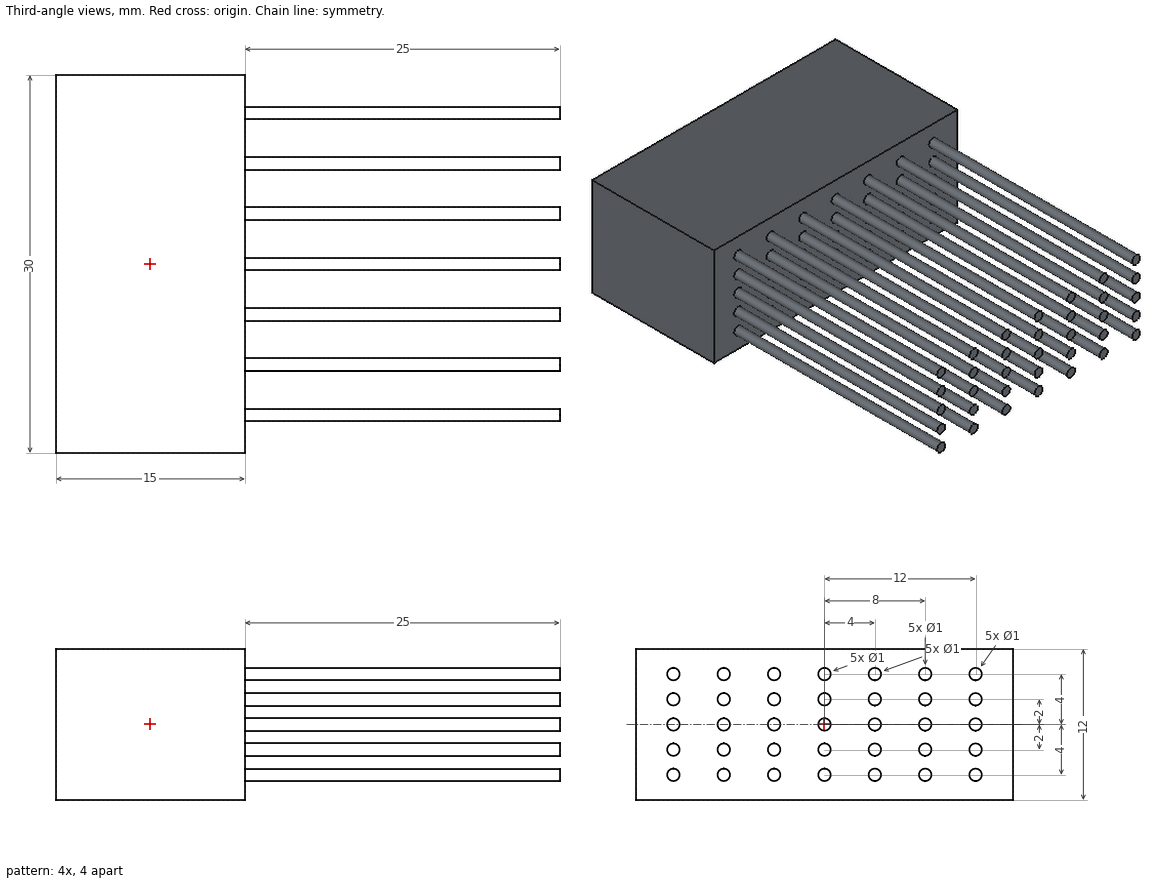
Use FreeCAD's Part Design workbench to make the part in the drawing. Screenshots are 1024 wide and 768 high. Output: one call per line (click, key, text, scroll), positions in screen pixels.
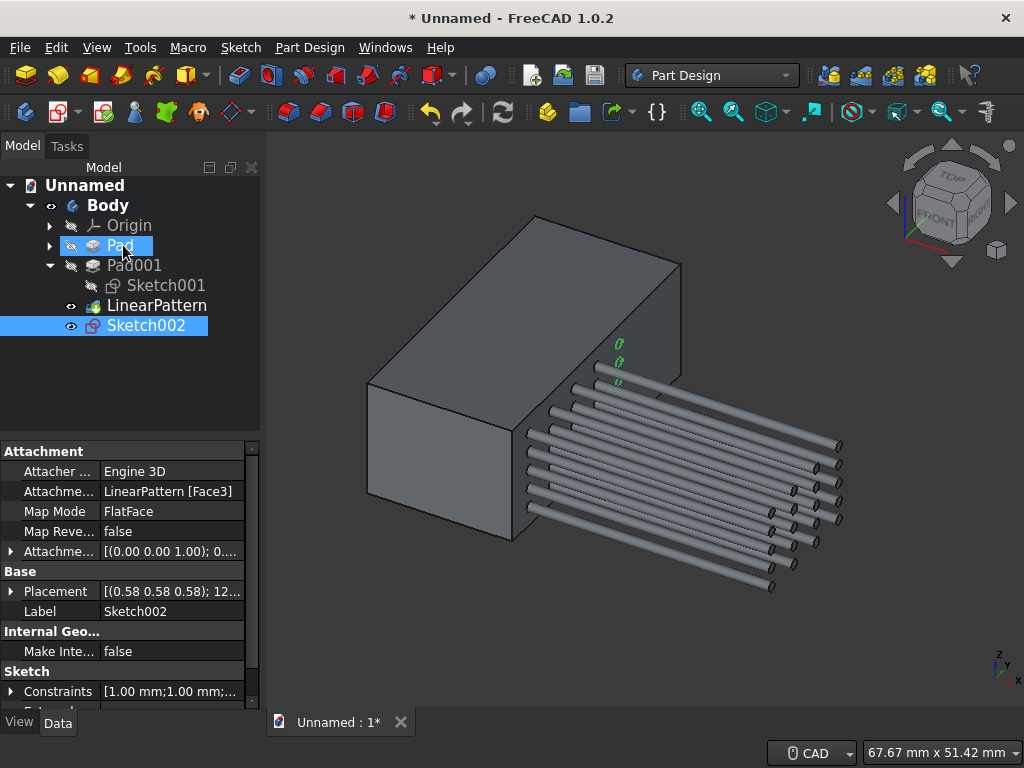
click(26, 76)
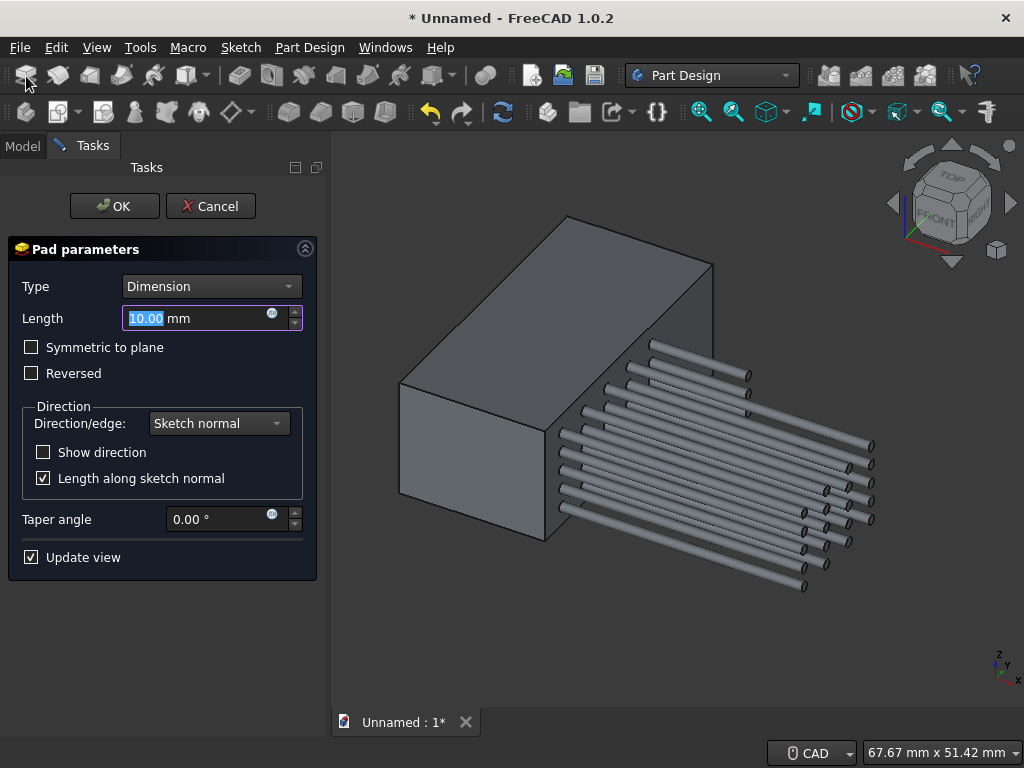
text(25)
key(Tab)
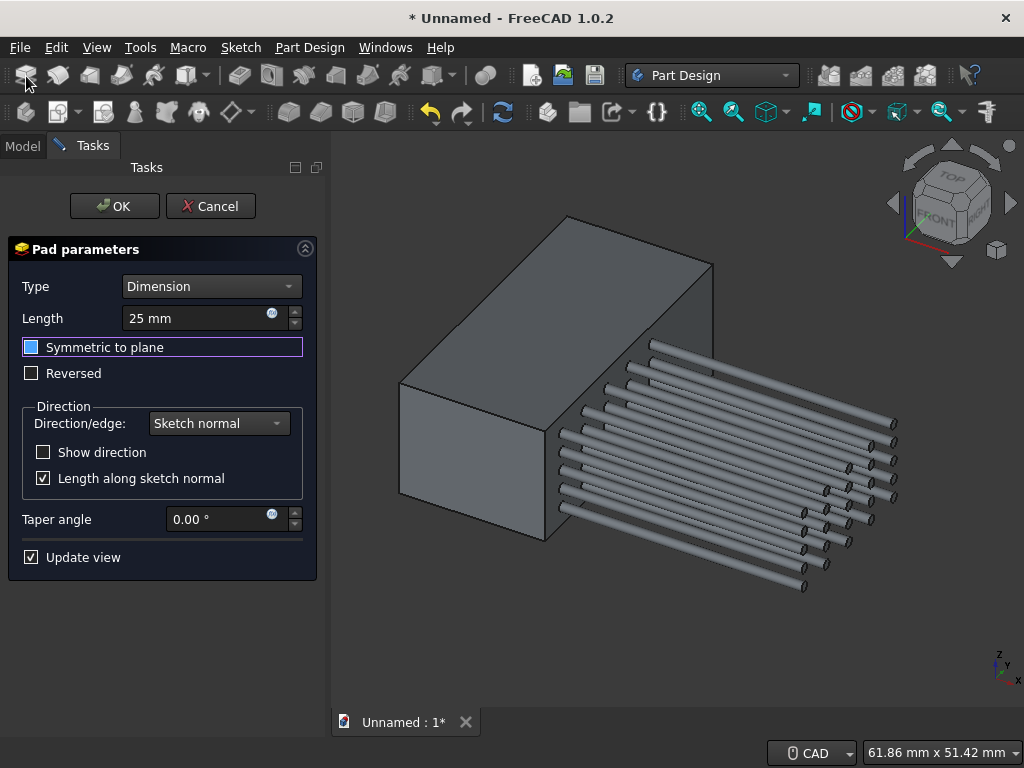
click(115, 206)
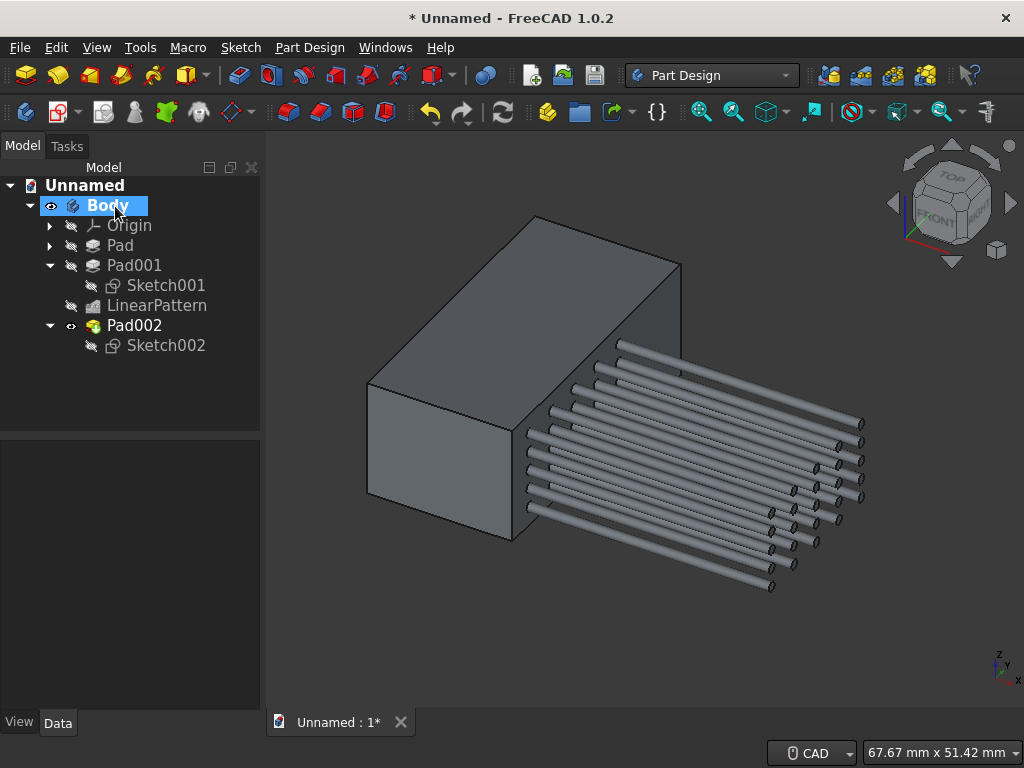
click(645, 323)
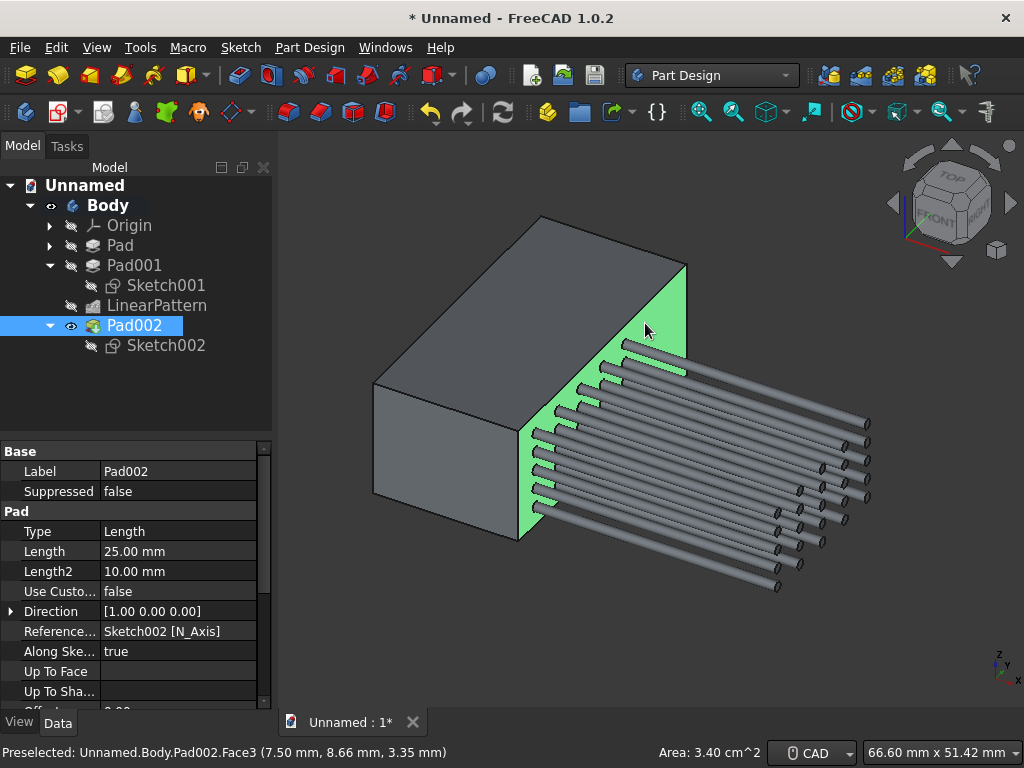
click(58, 112)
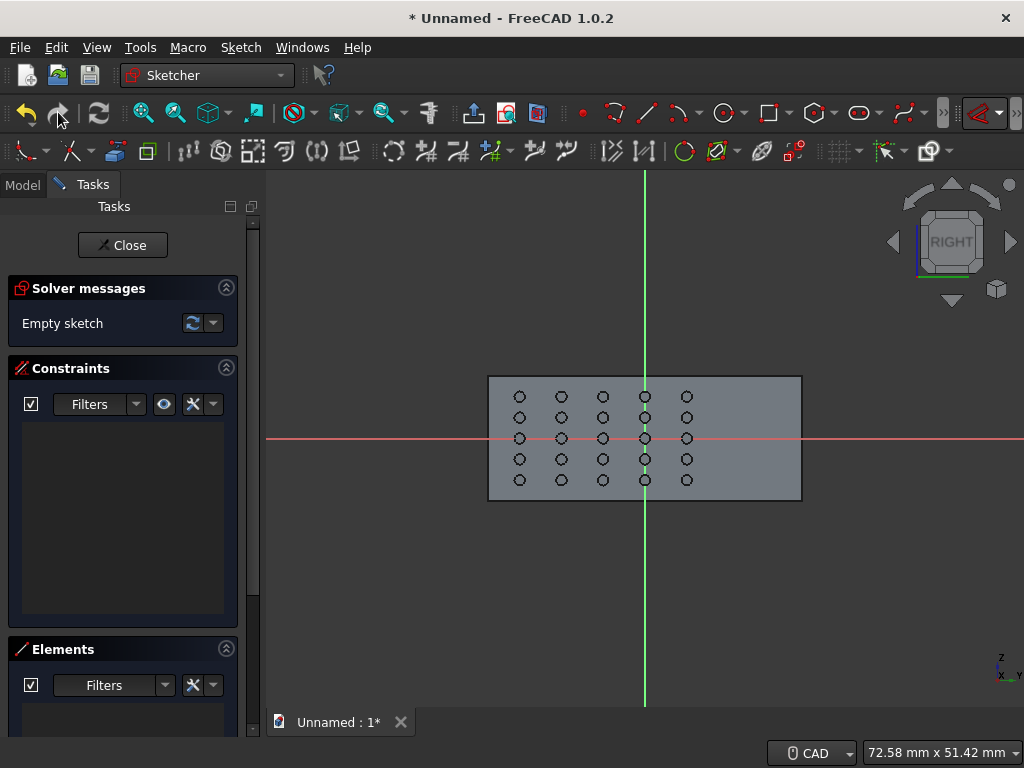
scroll(738, 438, up, 6)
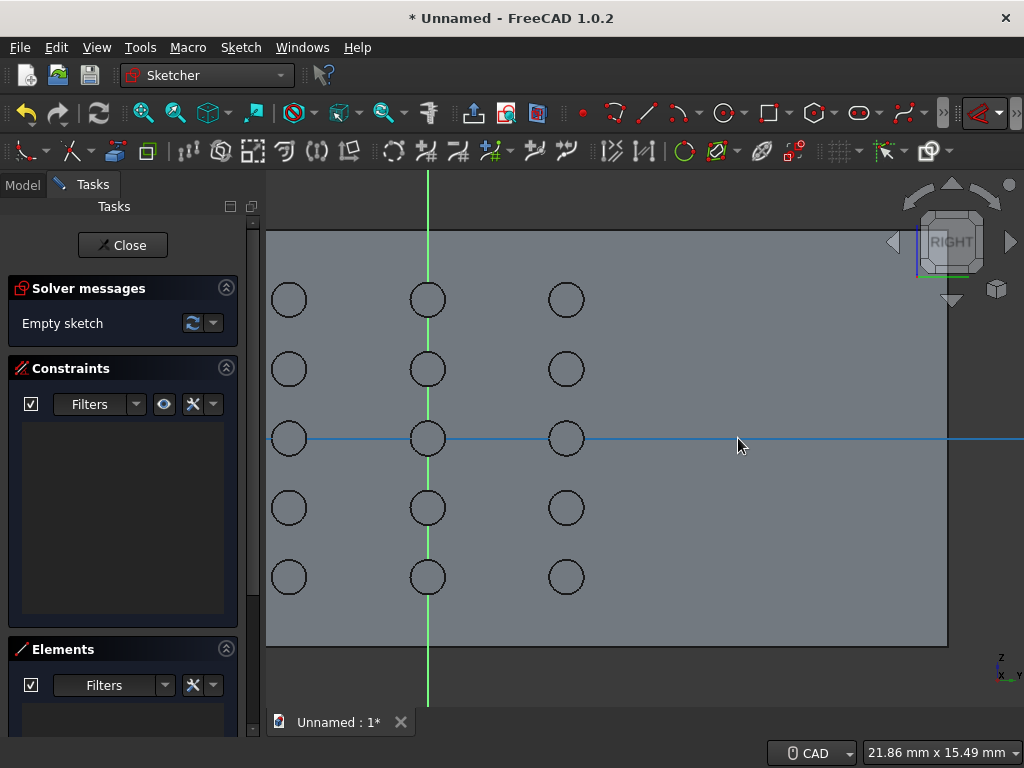
click(724, 114)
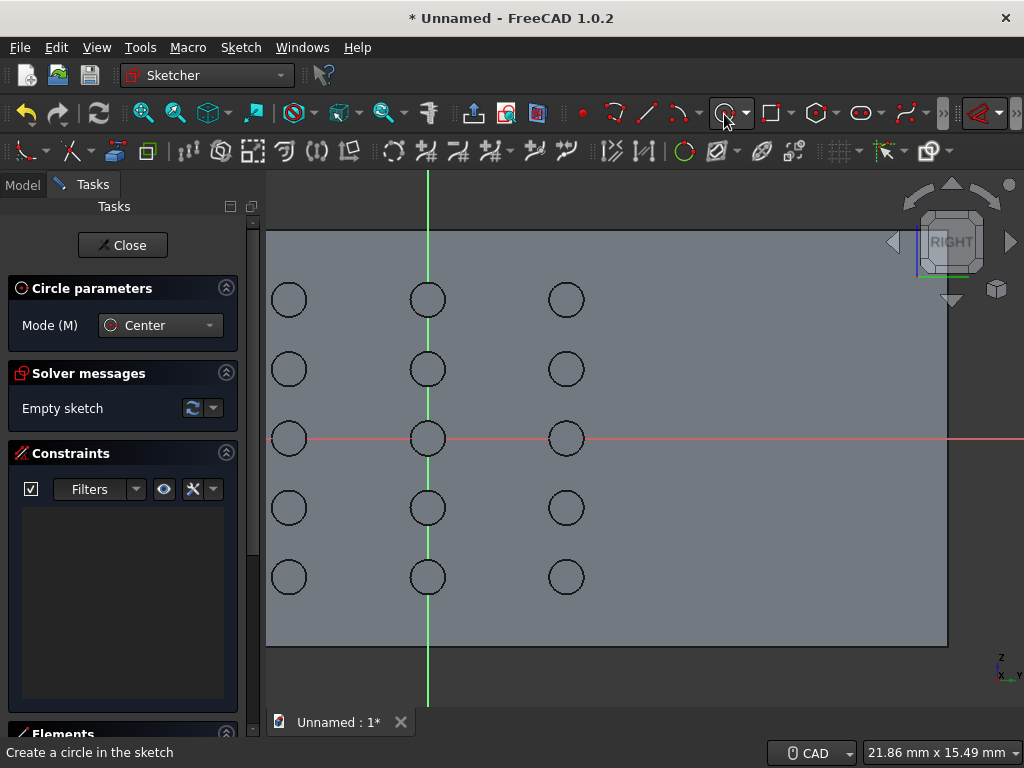
scroll(705, 300, up, 2)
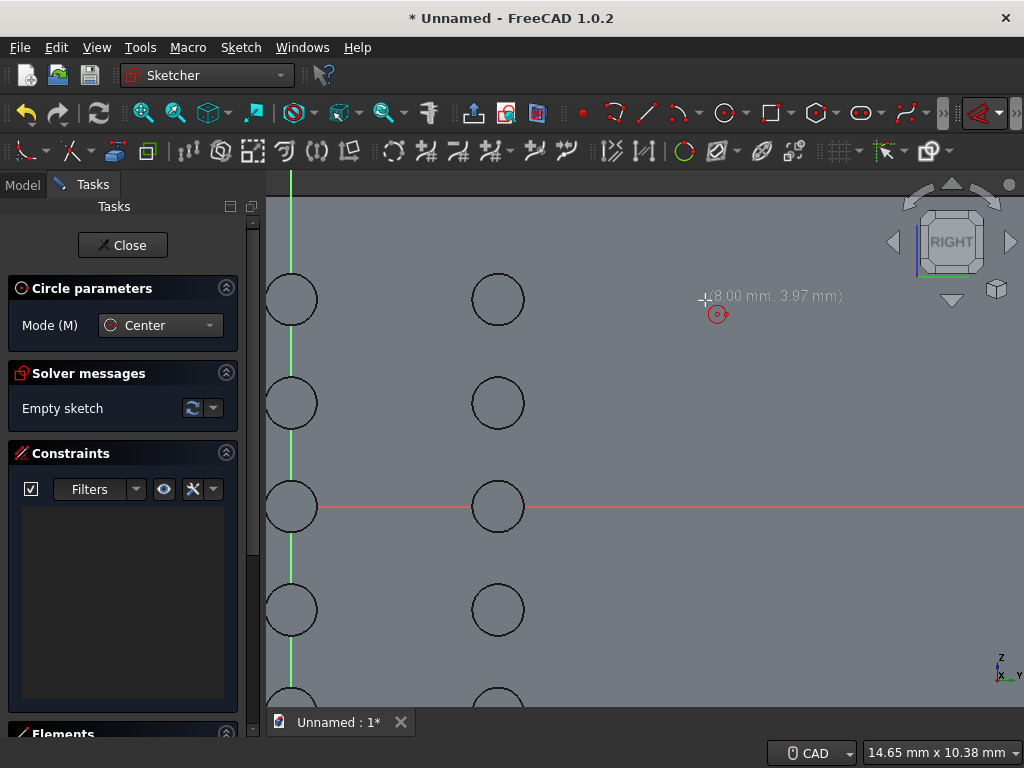
click(705, 300)
move(723, 281)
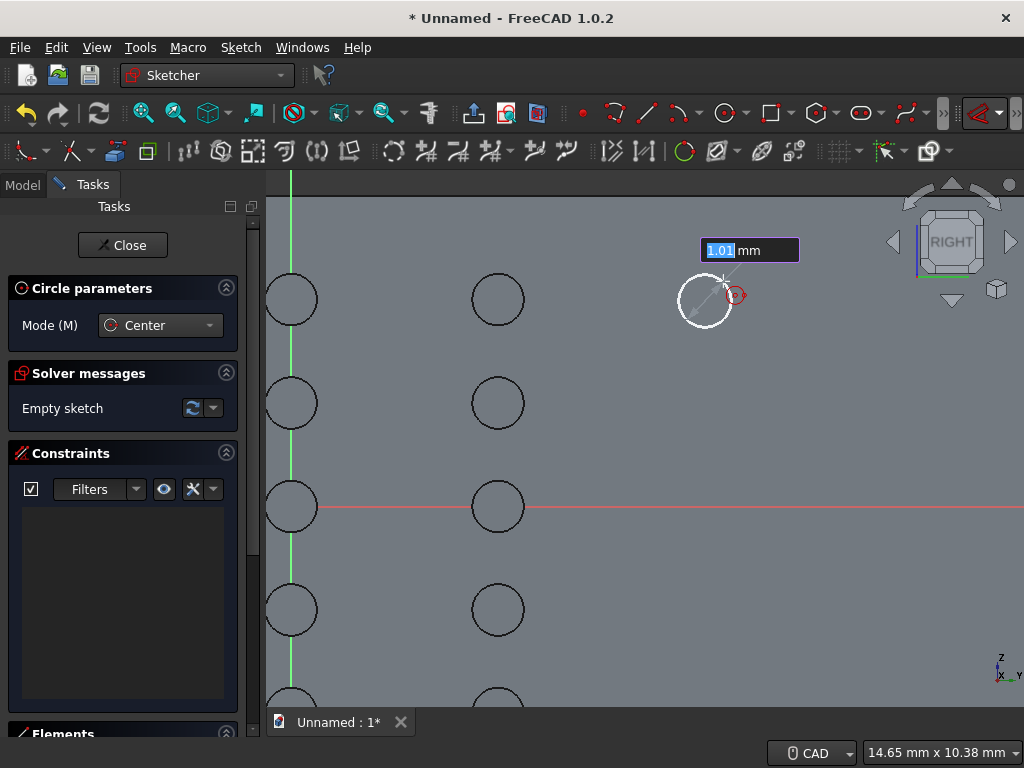
text(1)
key(Return)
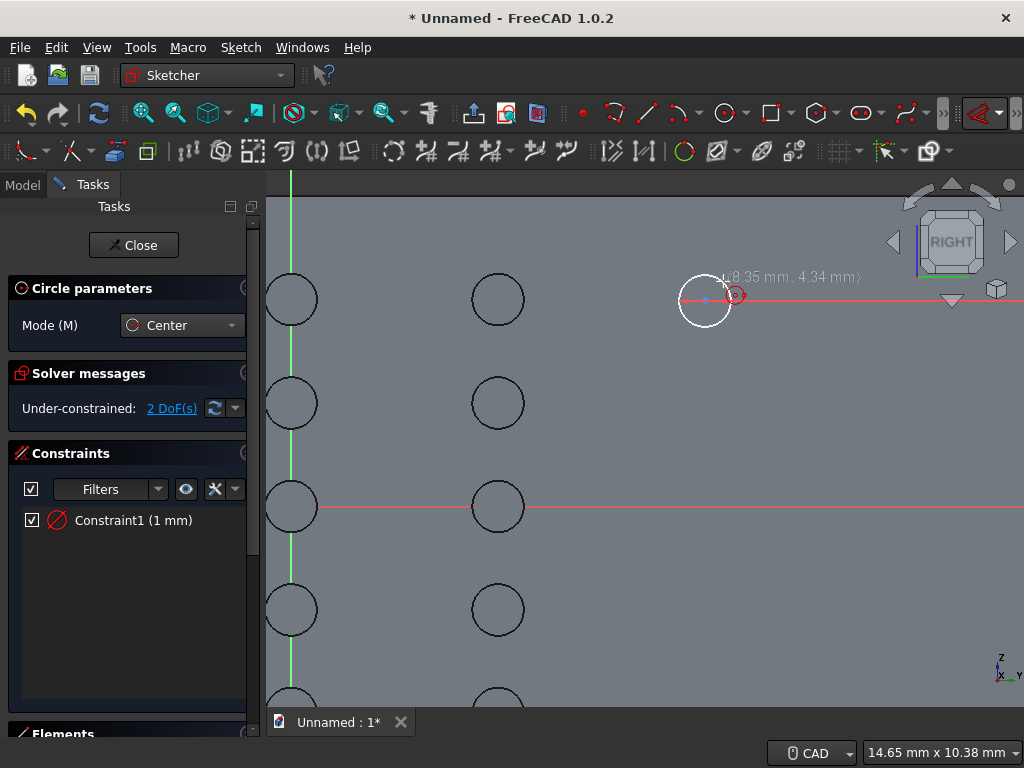
click(705, 403)
move(723, 385)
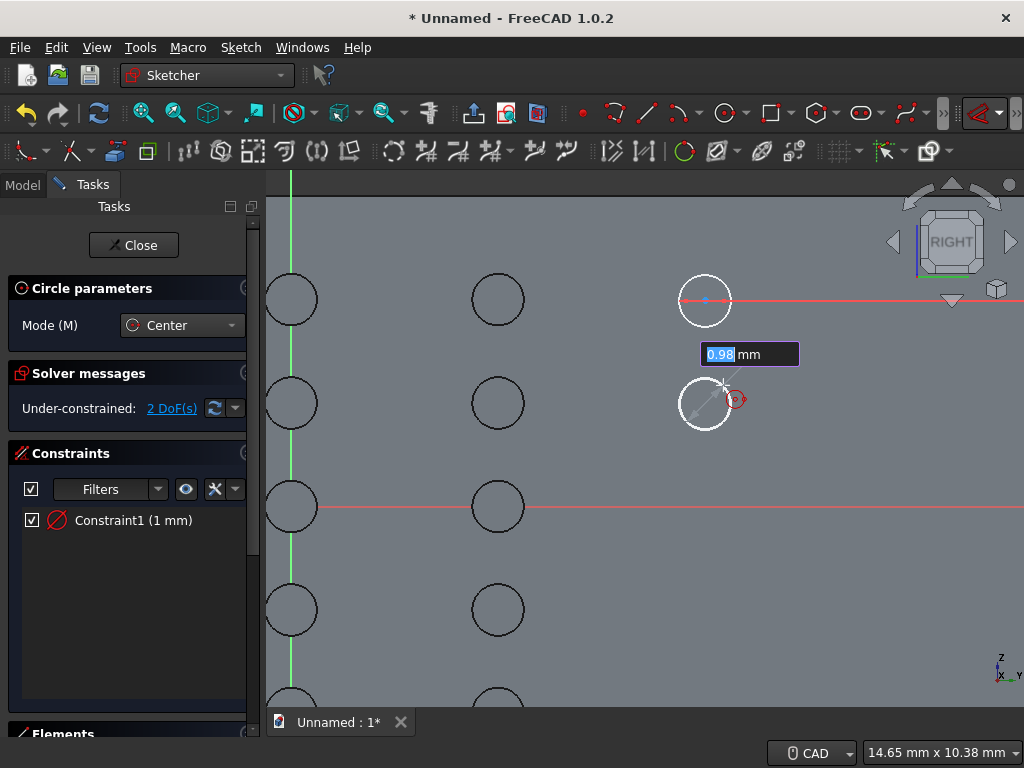
text(1)
key(Return)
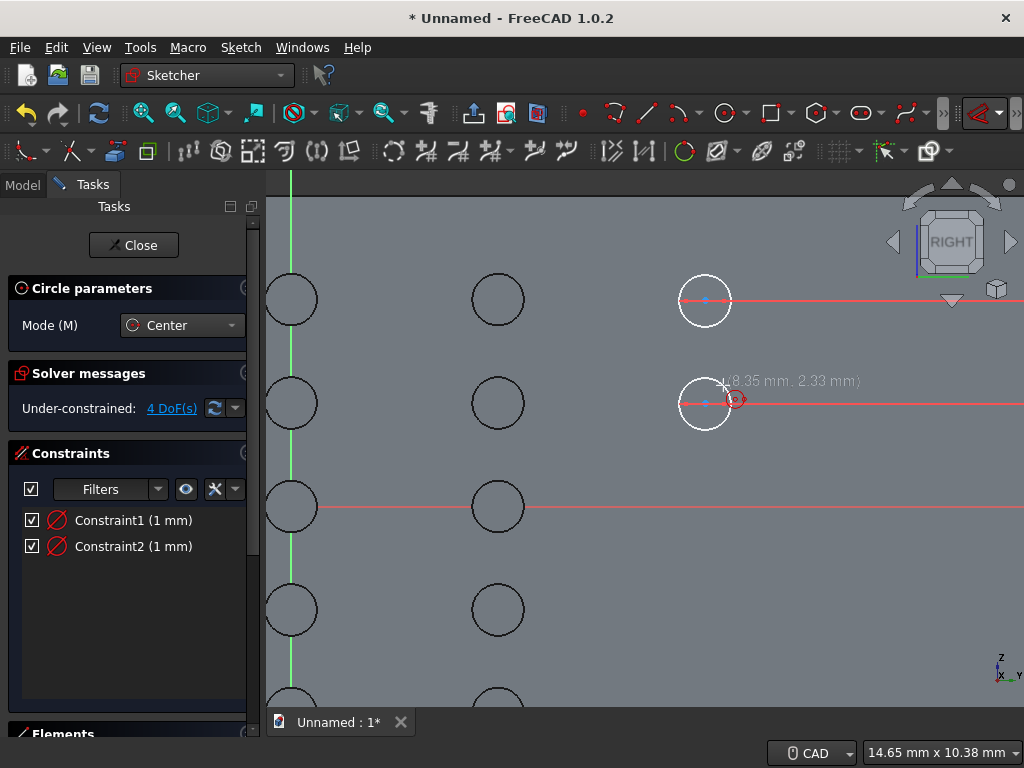
click(705, 506)
move(723, 488)